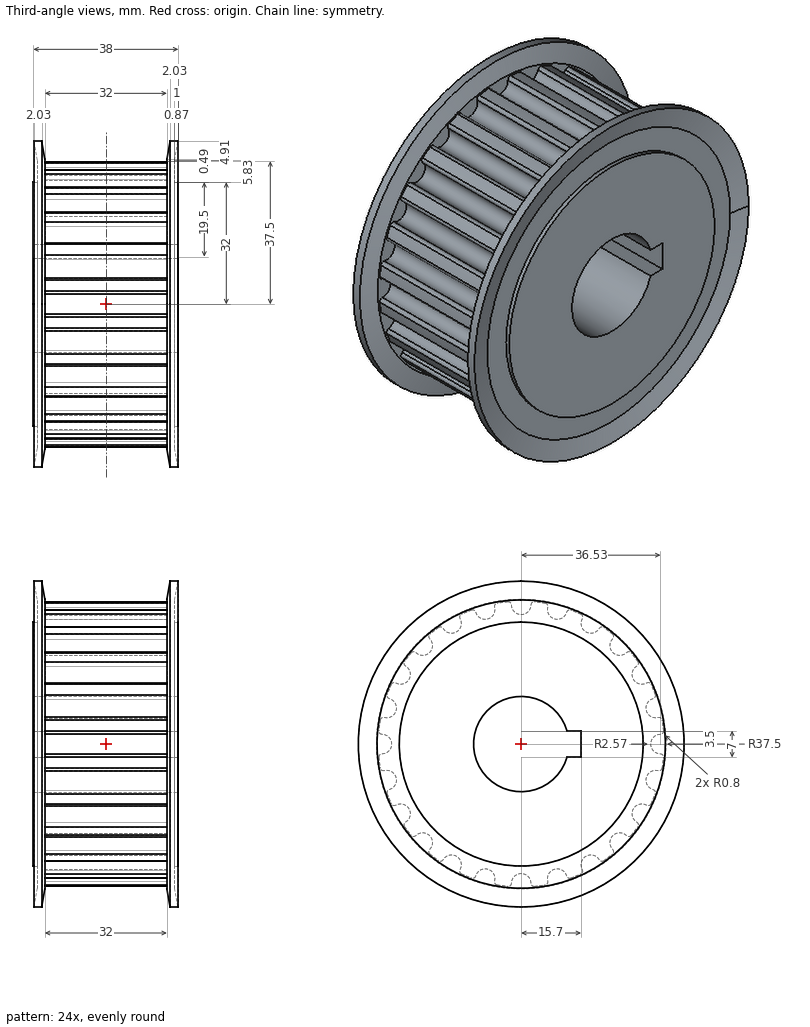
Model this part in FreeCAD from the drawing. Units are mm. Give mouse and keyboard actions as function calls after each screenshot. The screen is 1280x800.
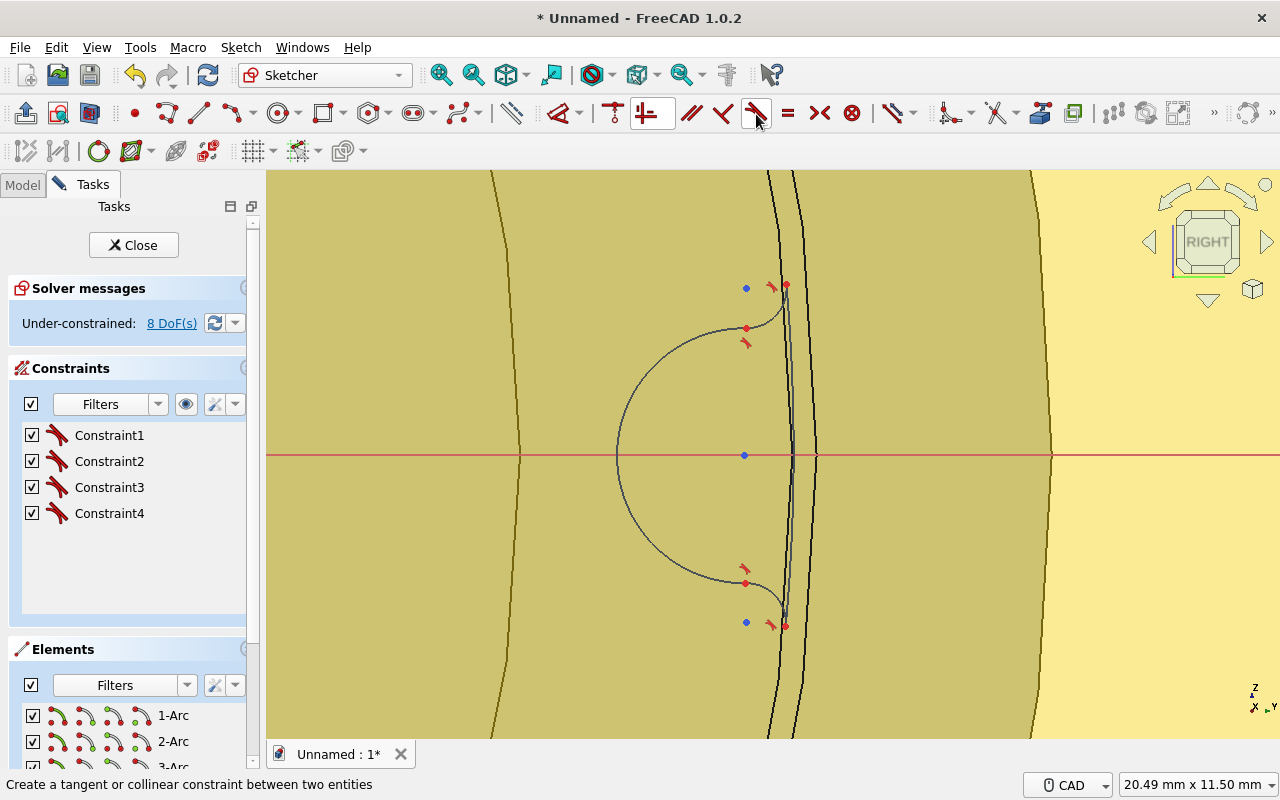
scroll(1075, 454, down, 6)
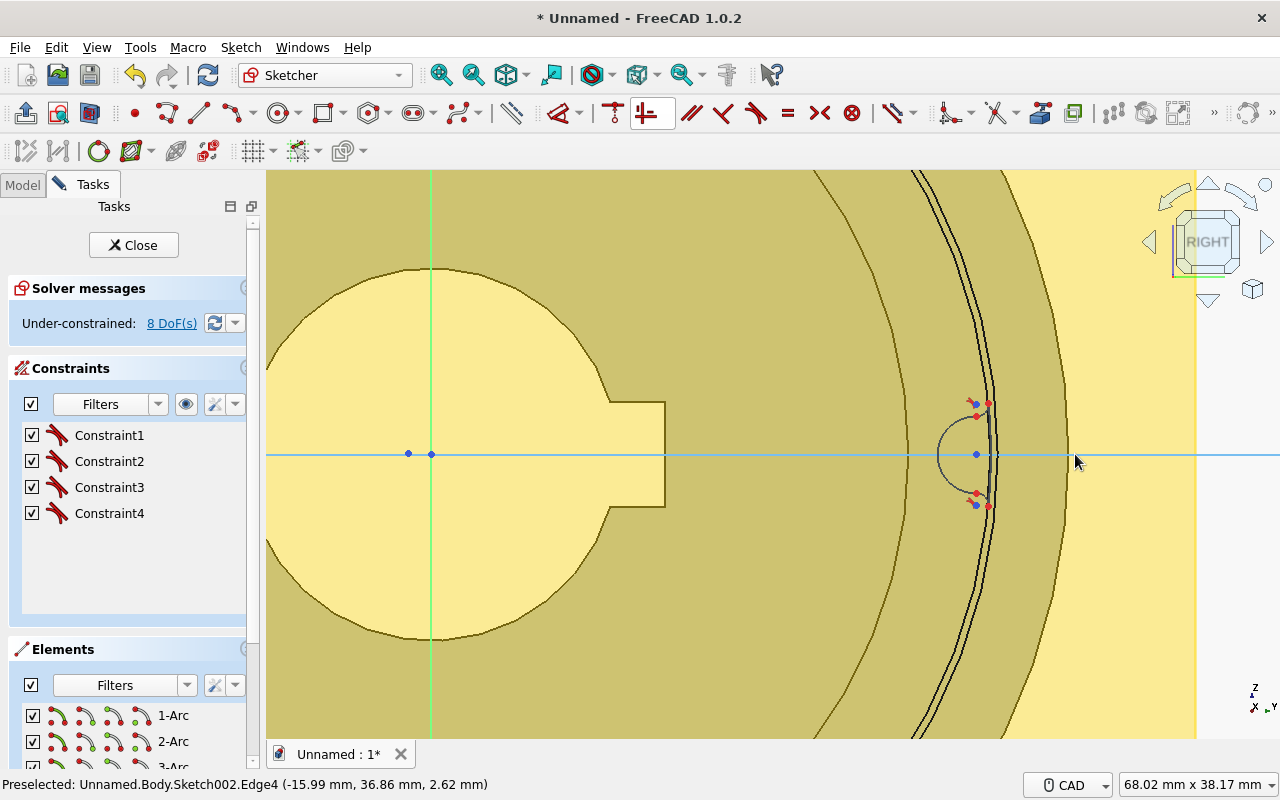
scroll(420, 454, up, 7)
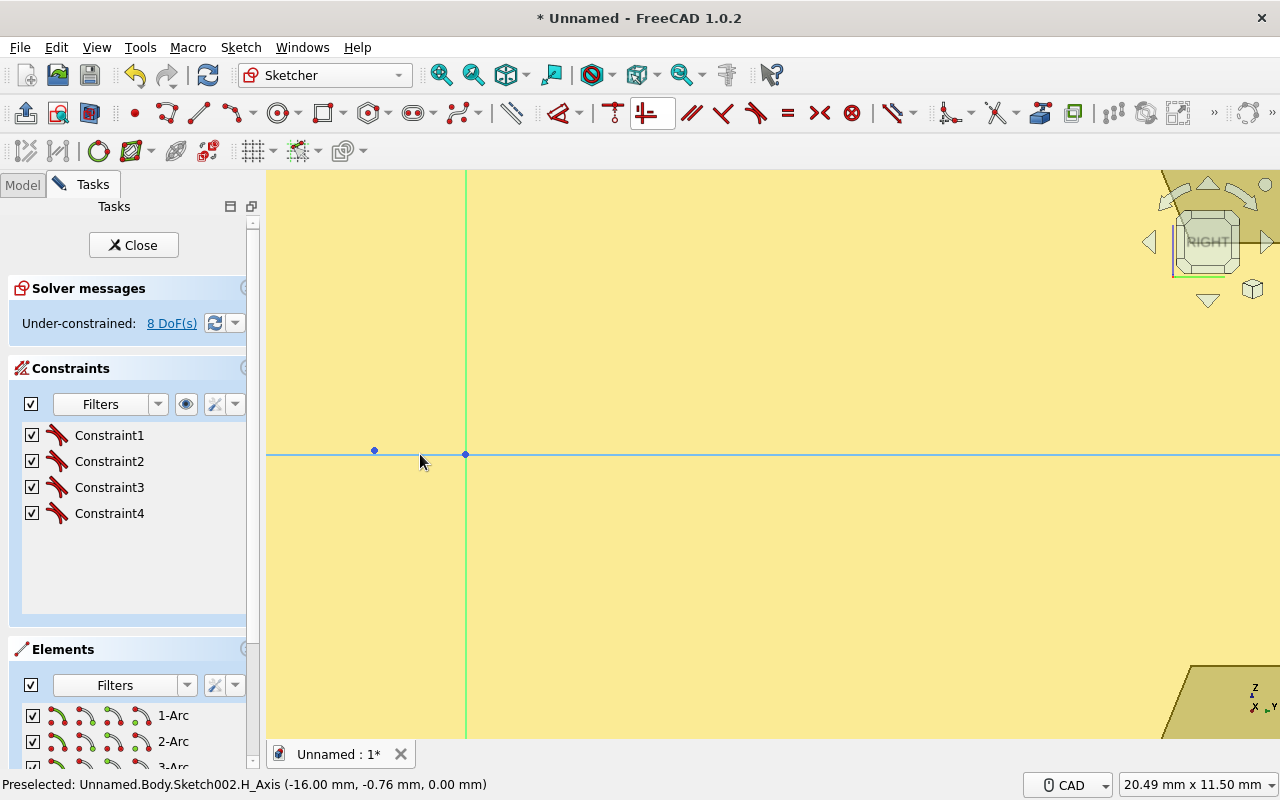
drag(365, 441, 476, 465)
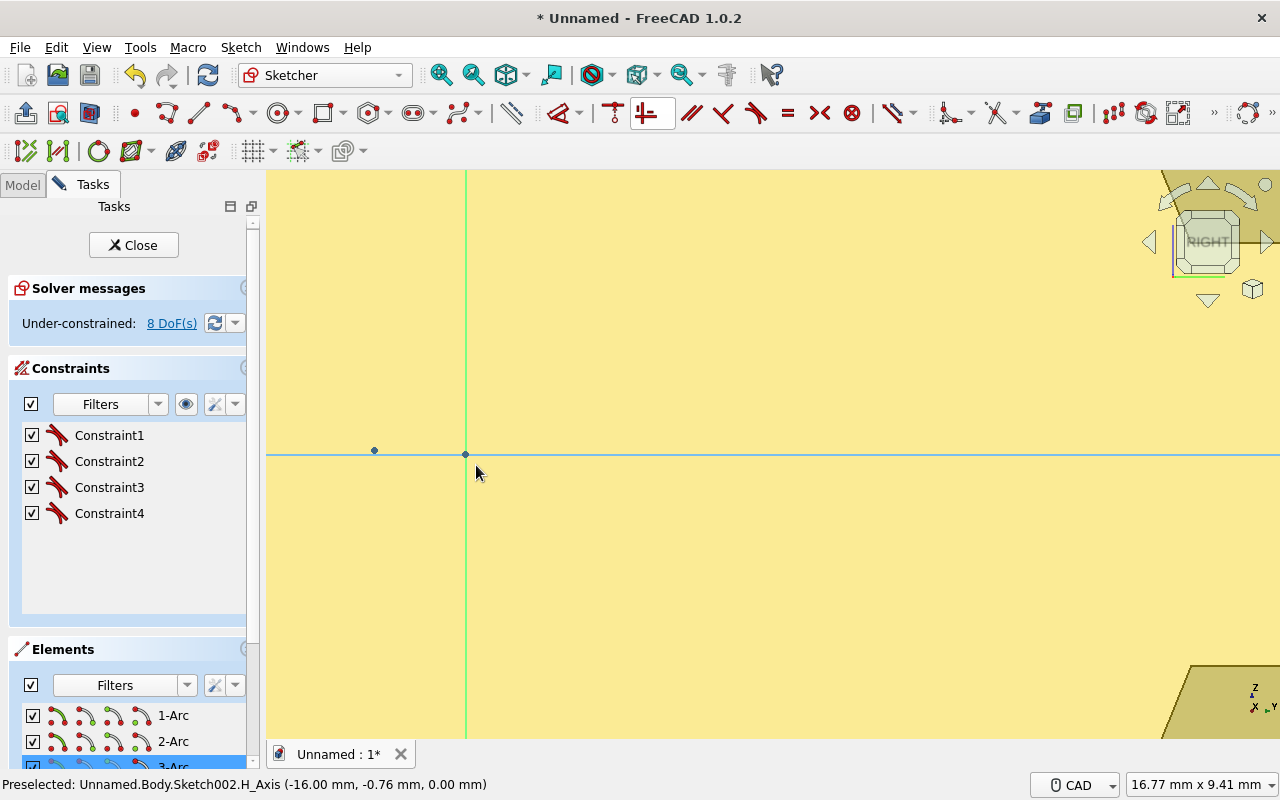
click(614, 114)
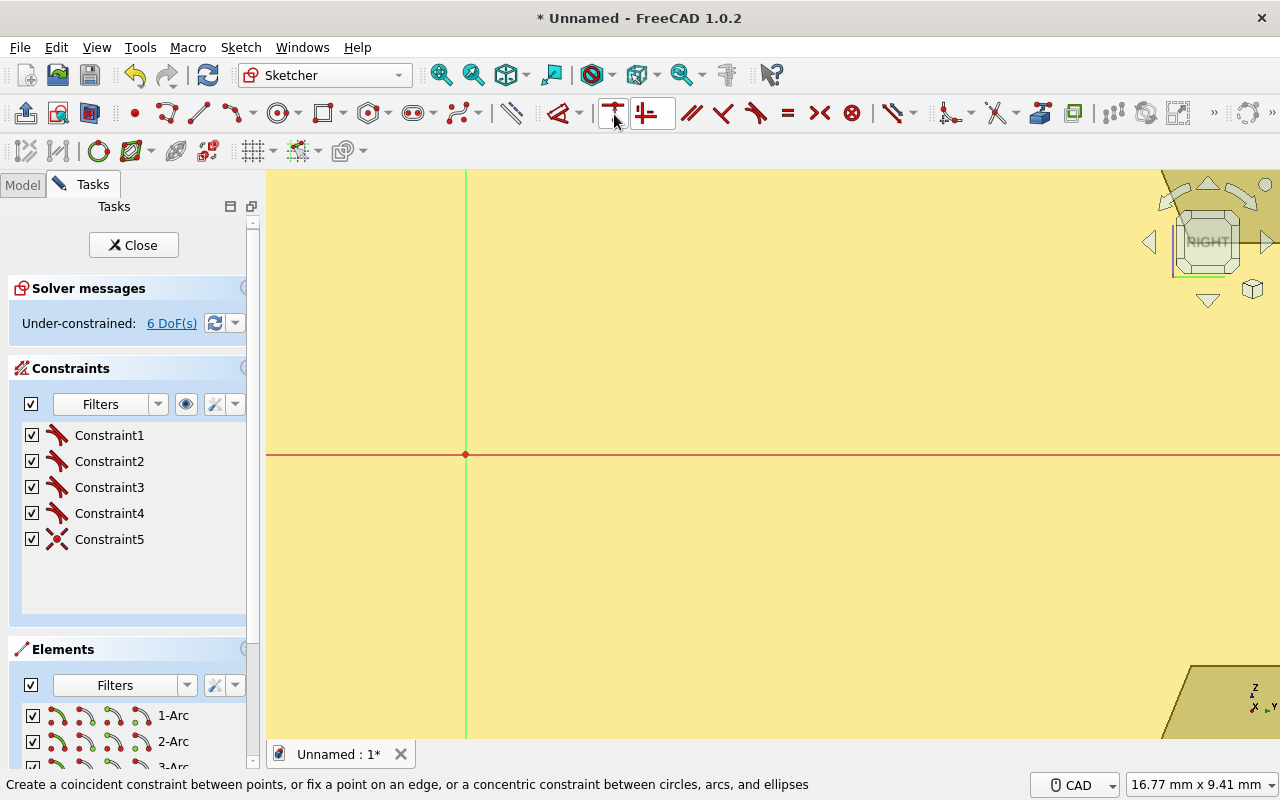
scroll(704, 454, down, 5)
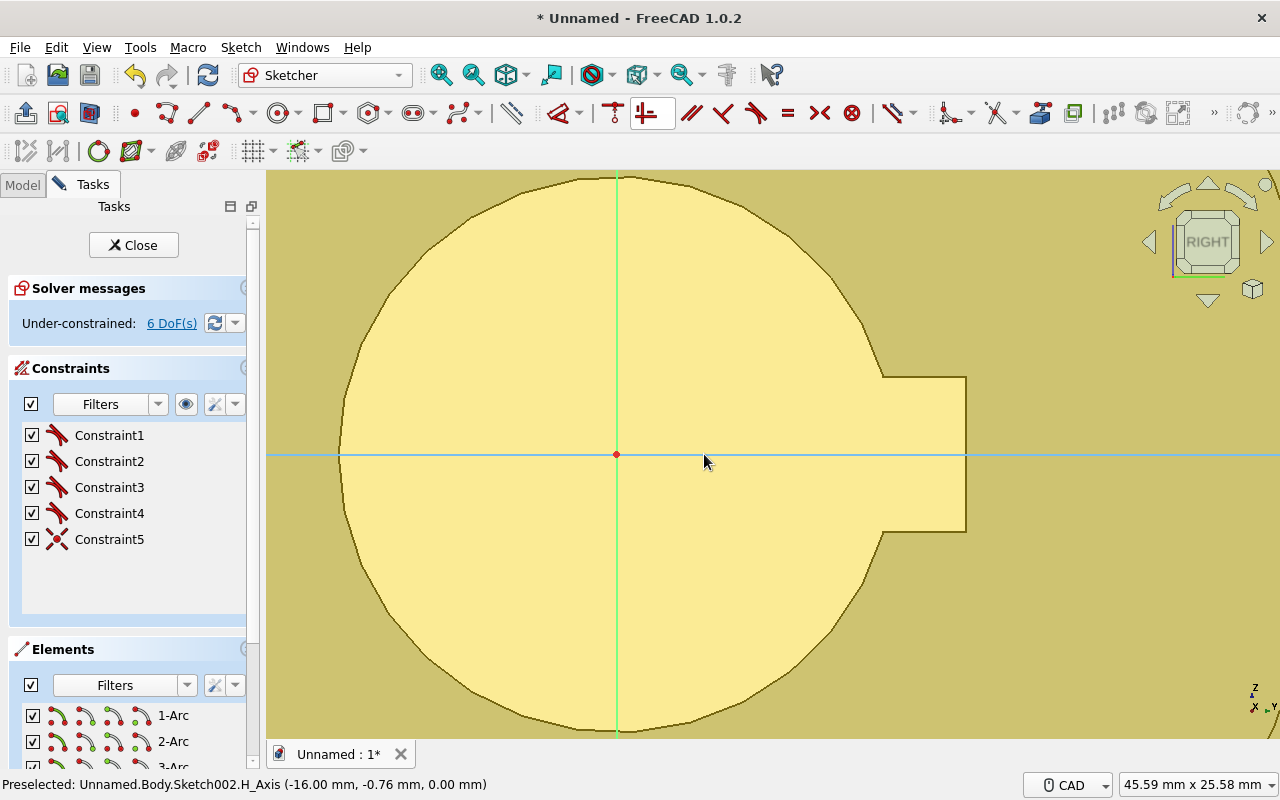
scroll(704, 454, down, 5)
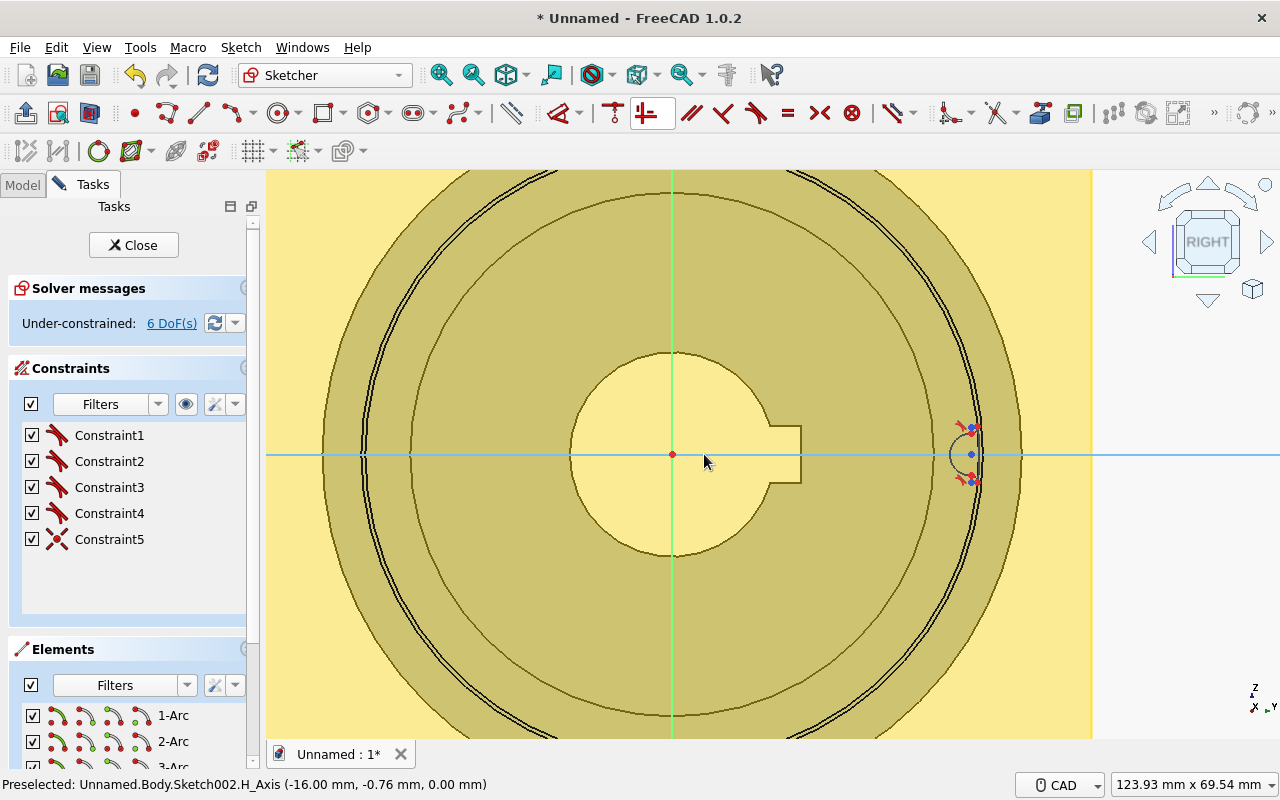
scroll(1016, 455, up, 9)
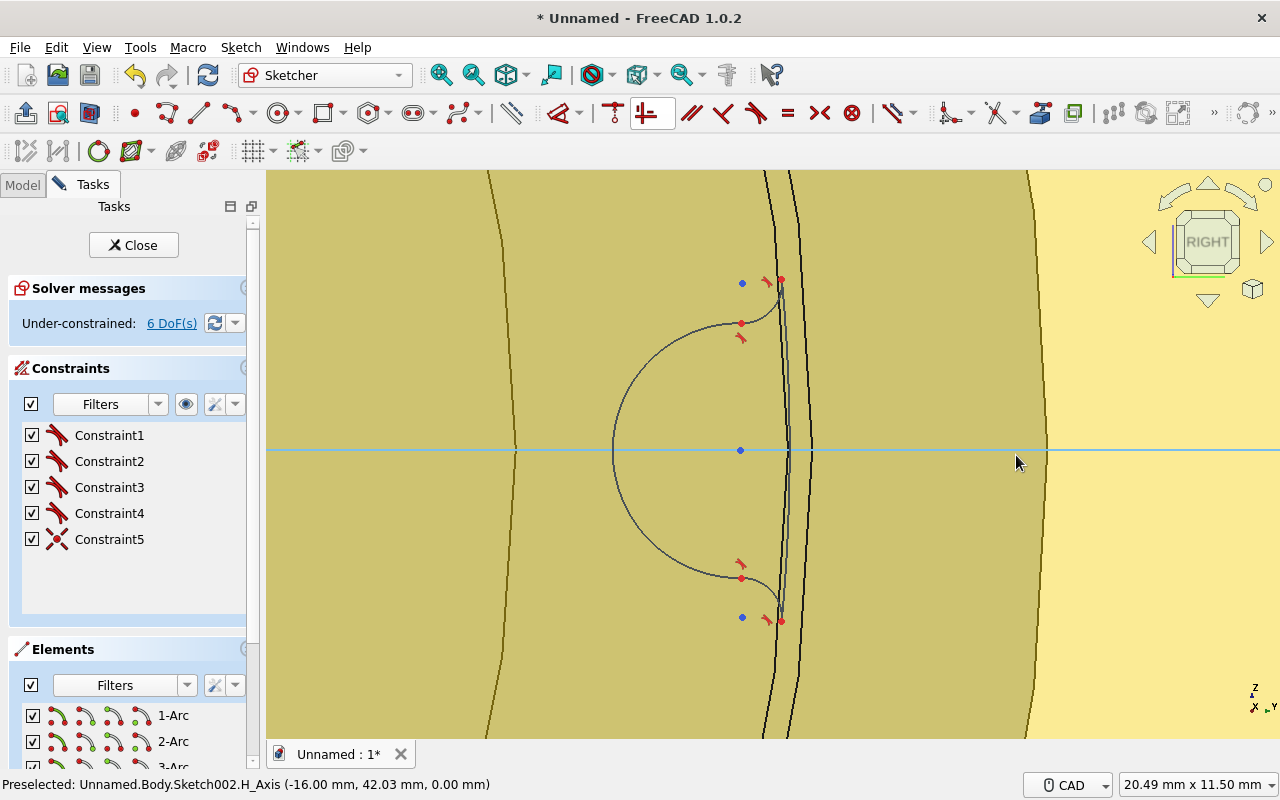
click(761, 583)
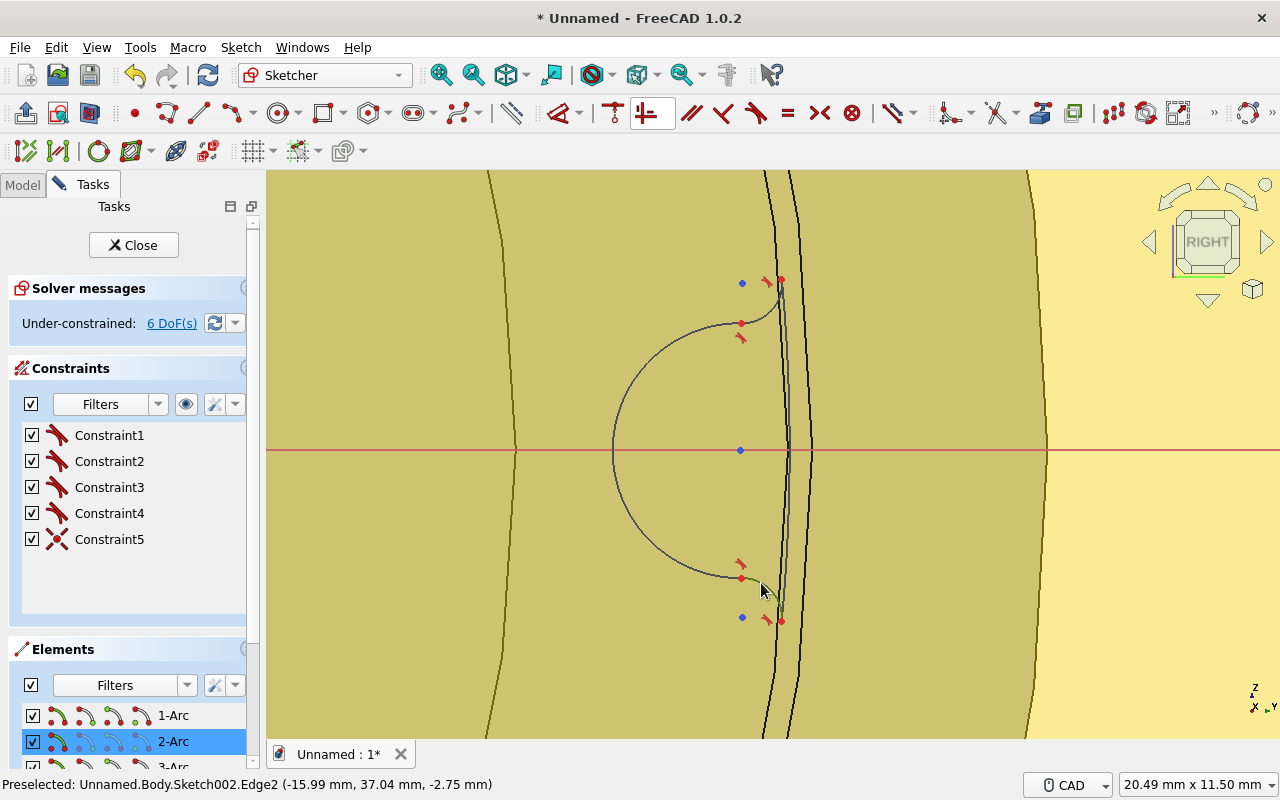
click(761, 319)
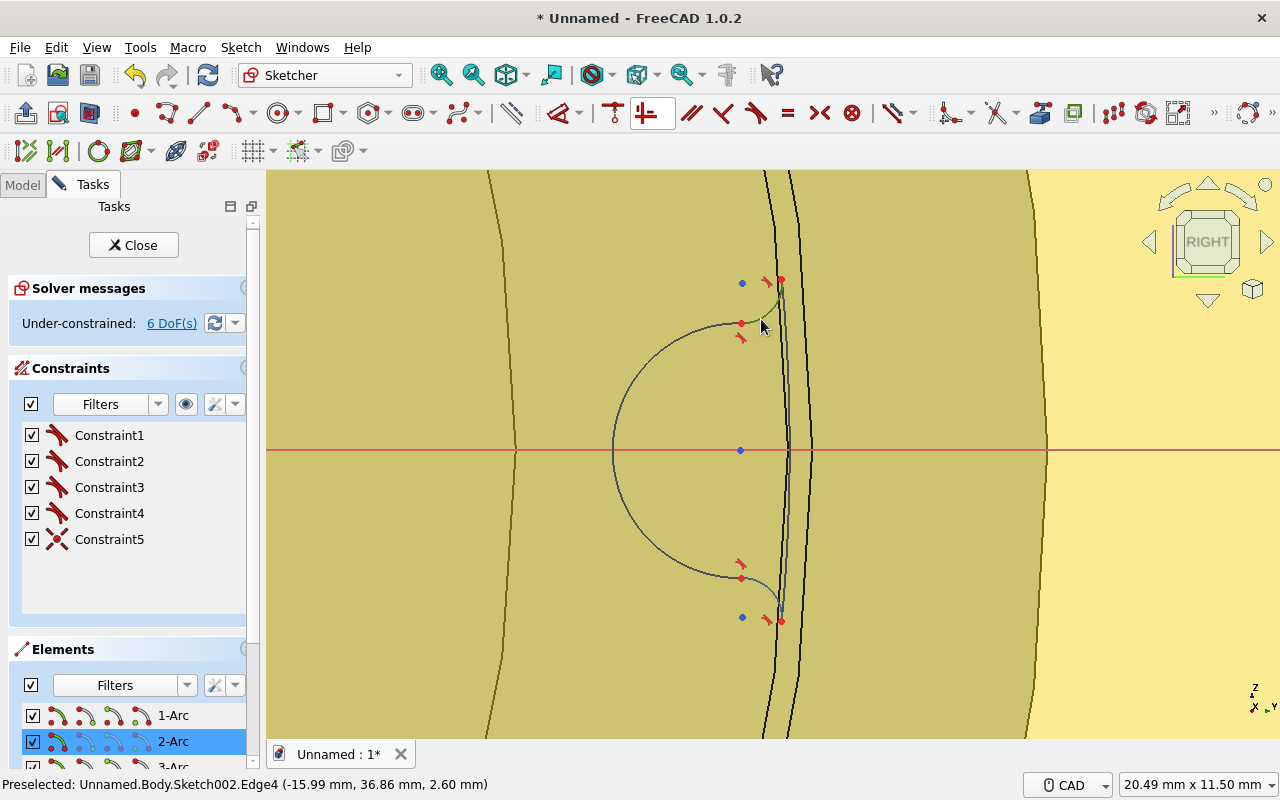
click(788, 114)